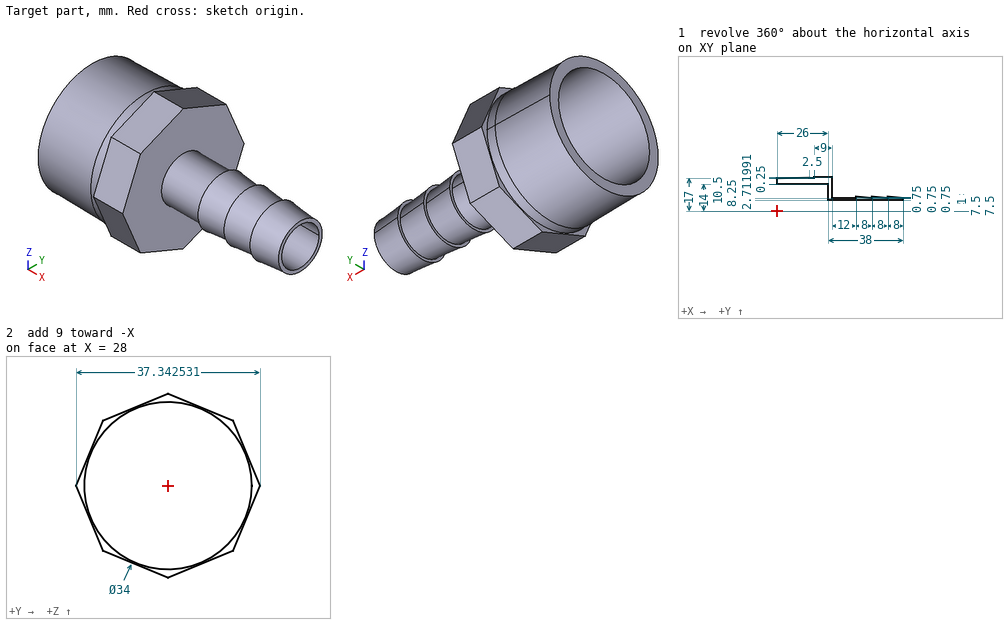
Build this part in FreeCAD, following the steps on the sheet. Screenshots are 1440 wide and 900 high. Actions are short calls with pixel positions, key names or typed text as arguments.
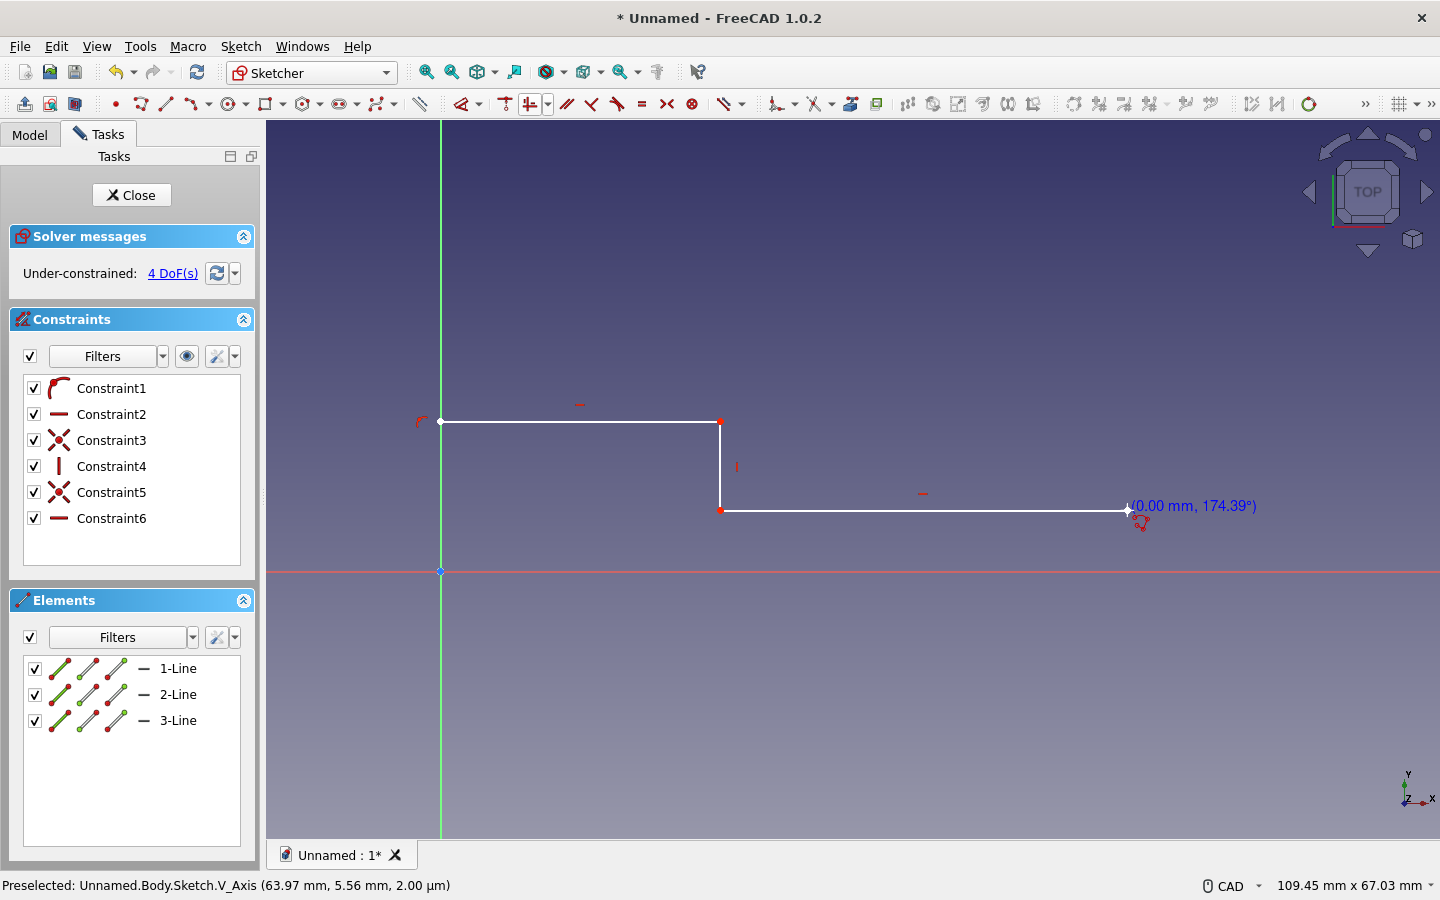
scroll(1127, 499, up, 2)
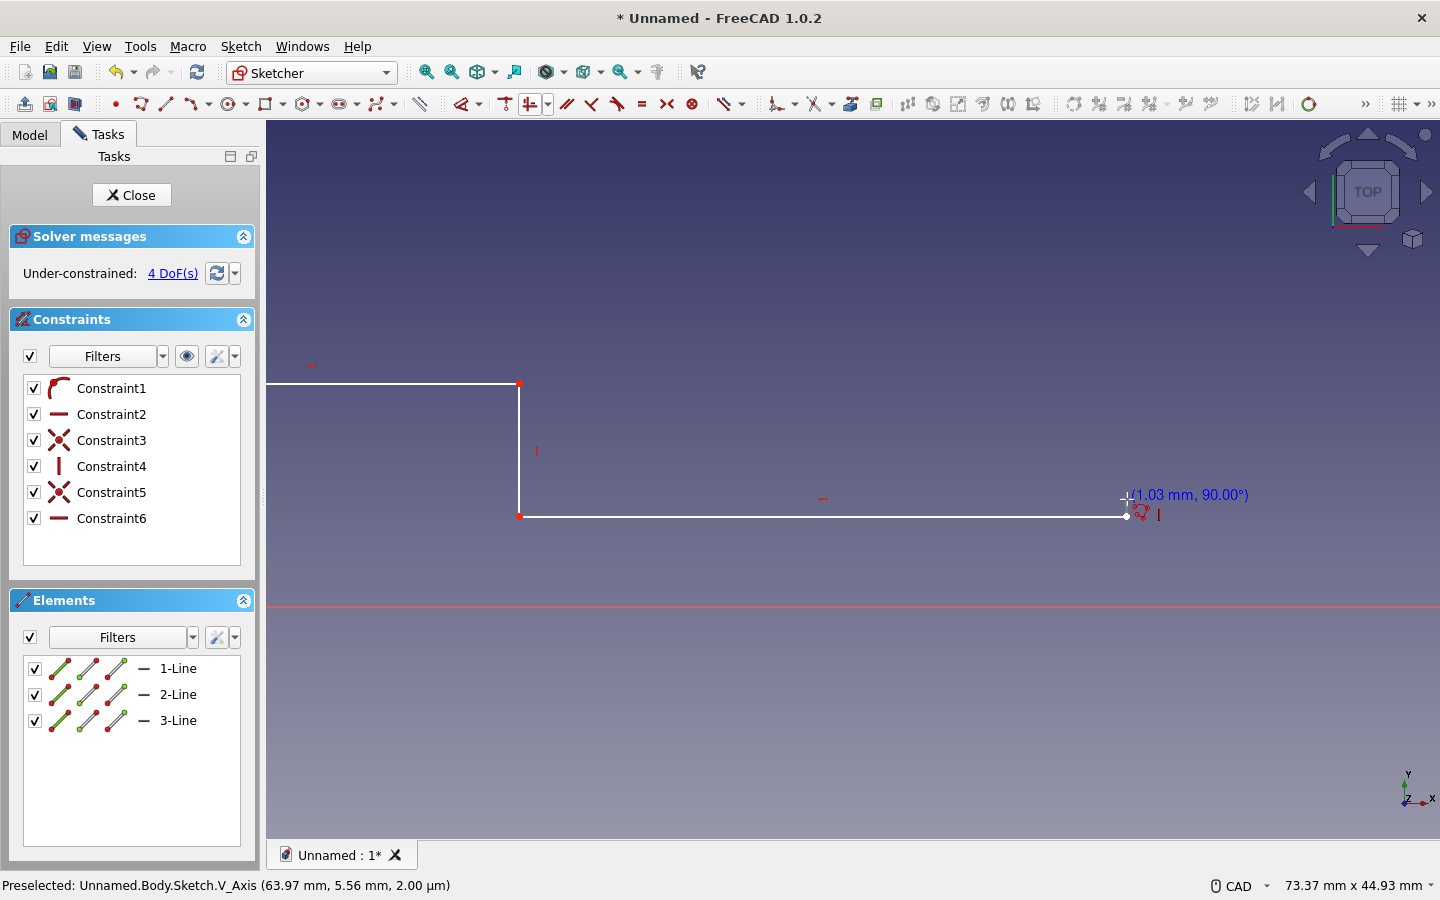
click(1127, 499)
click(999, 487)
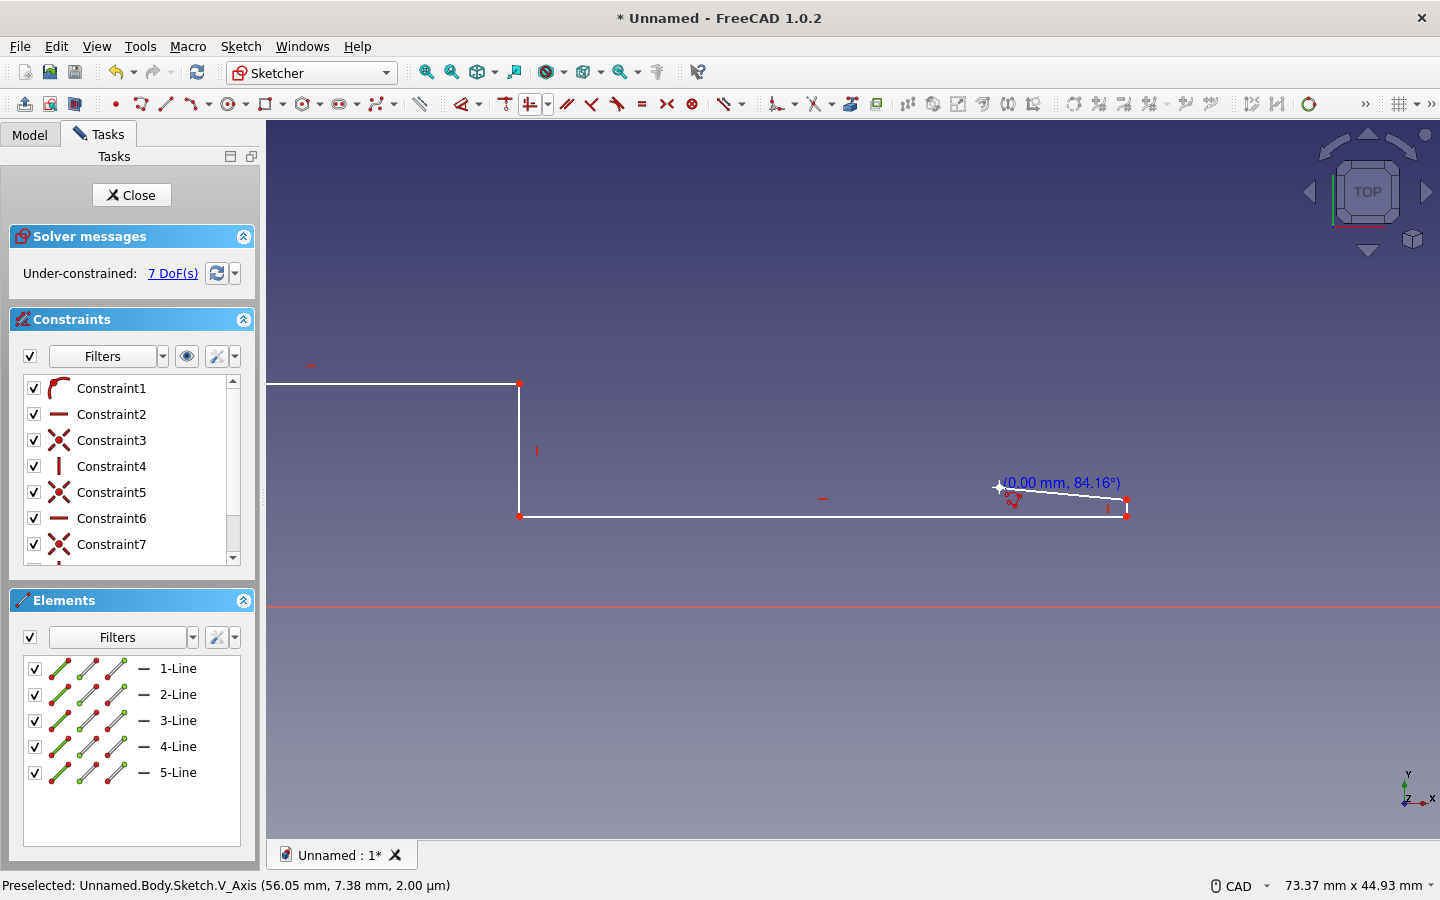
scroll(999, 499, up, 2)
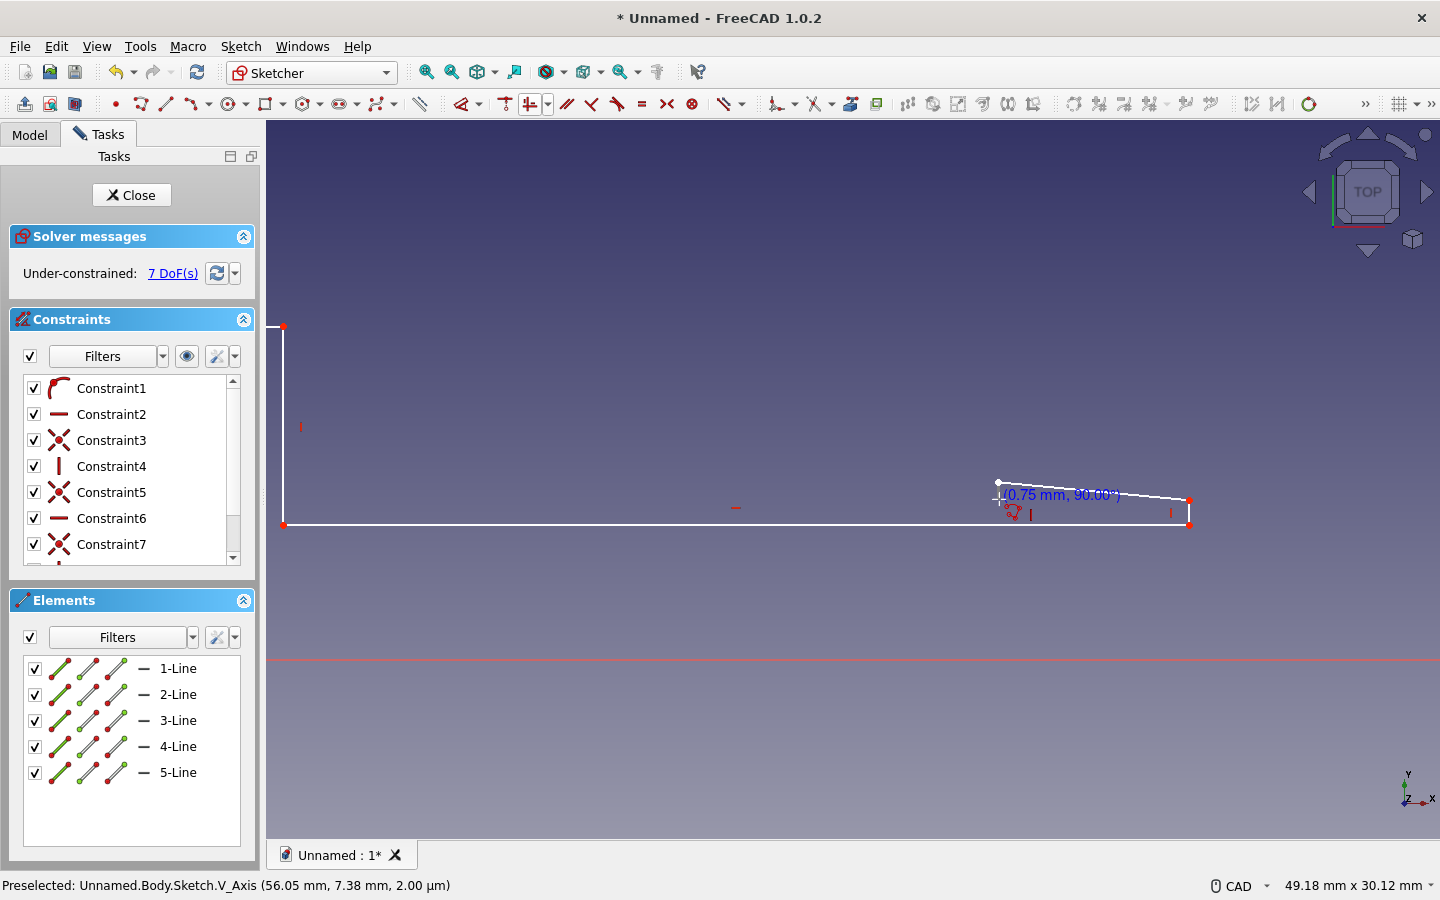
click(999, 499)
click(808, 481)
click(808, 499)
click(617, 481)
click(617, 499)
click(330, 499)
click(330, 248)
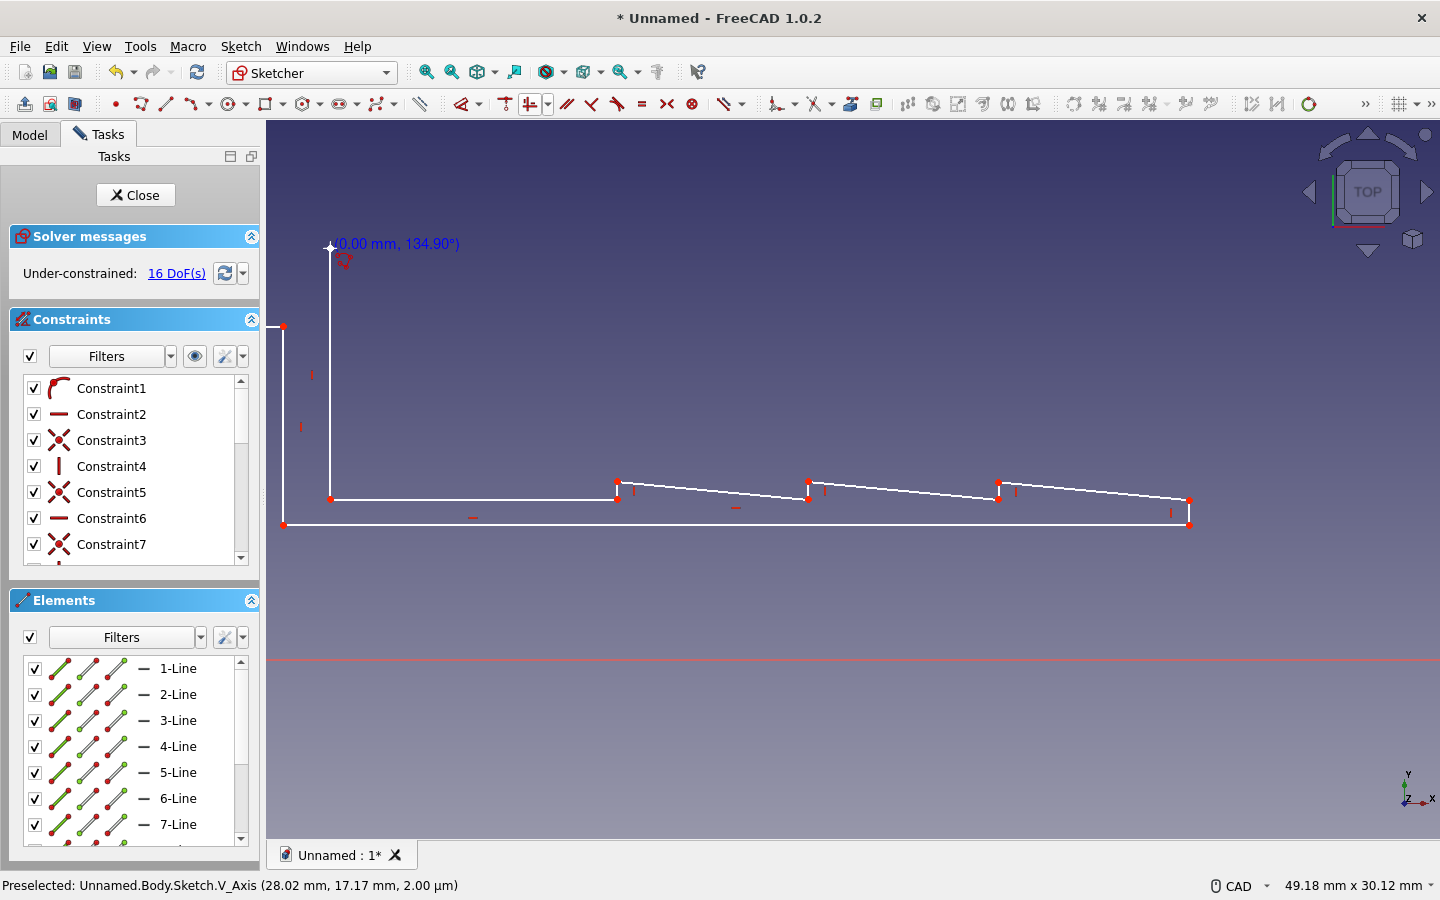
scroll(1077, 500, down, 4)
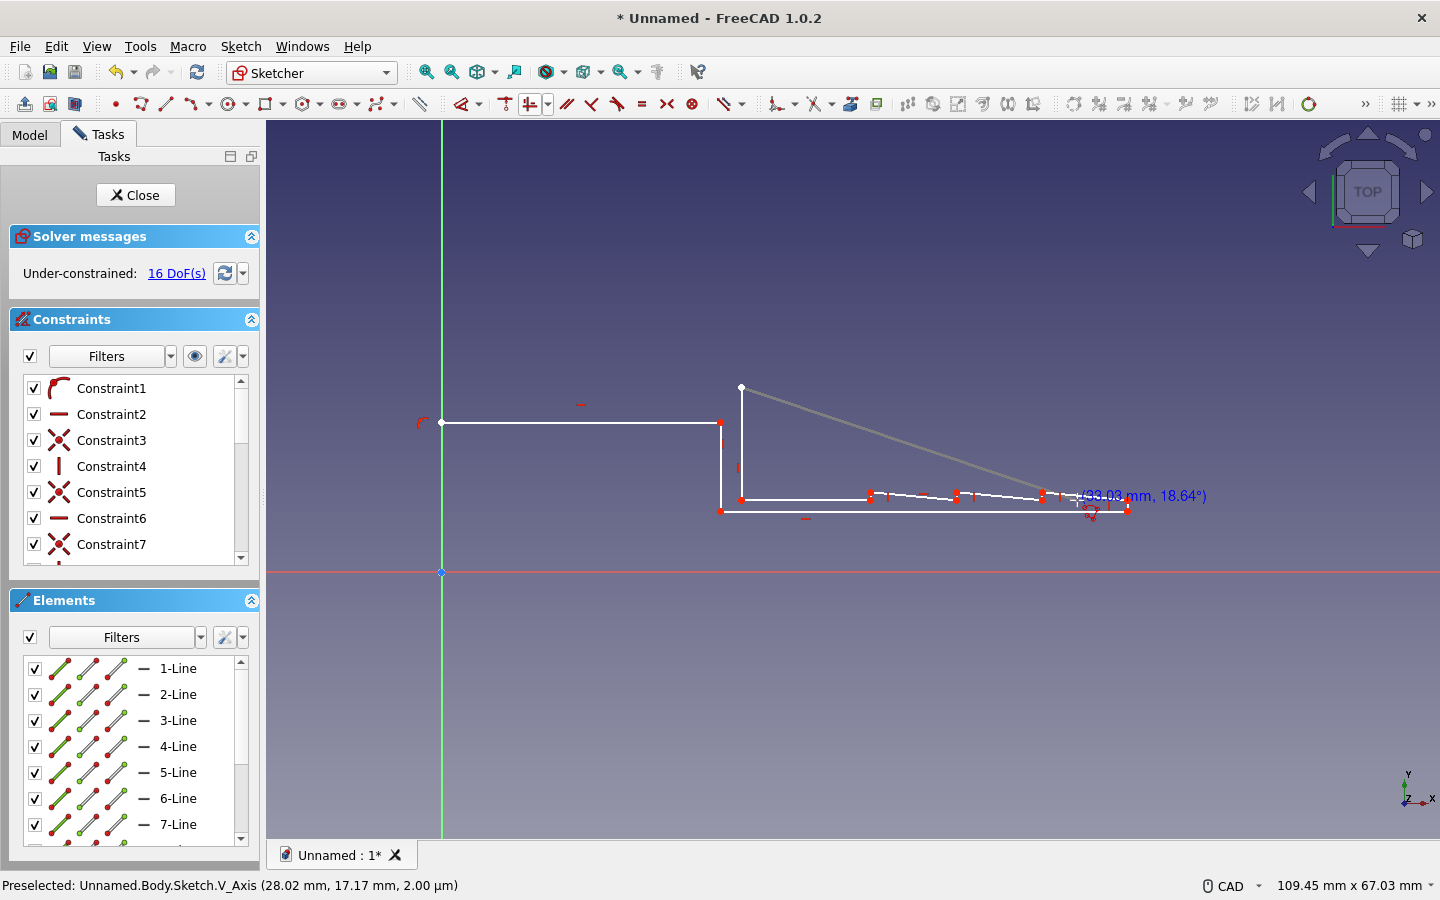
click(645, 387)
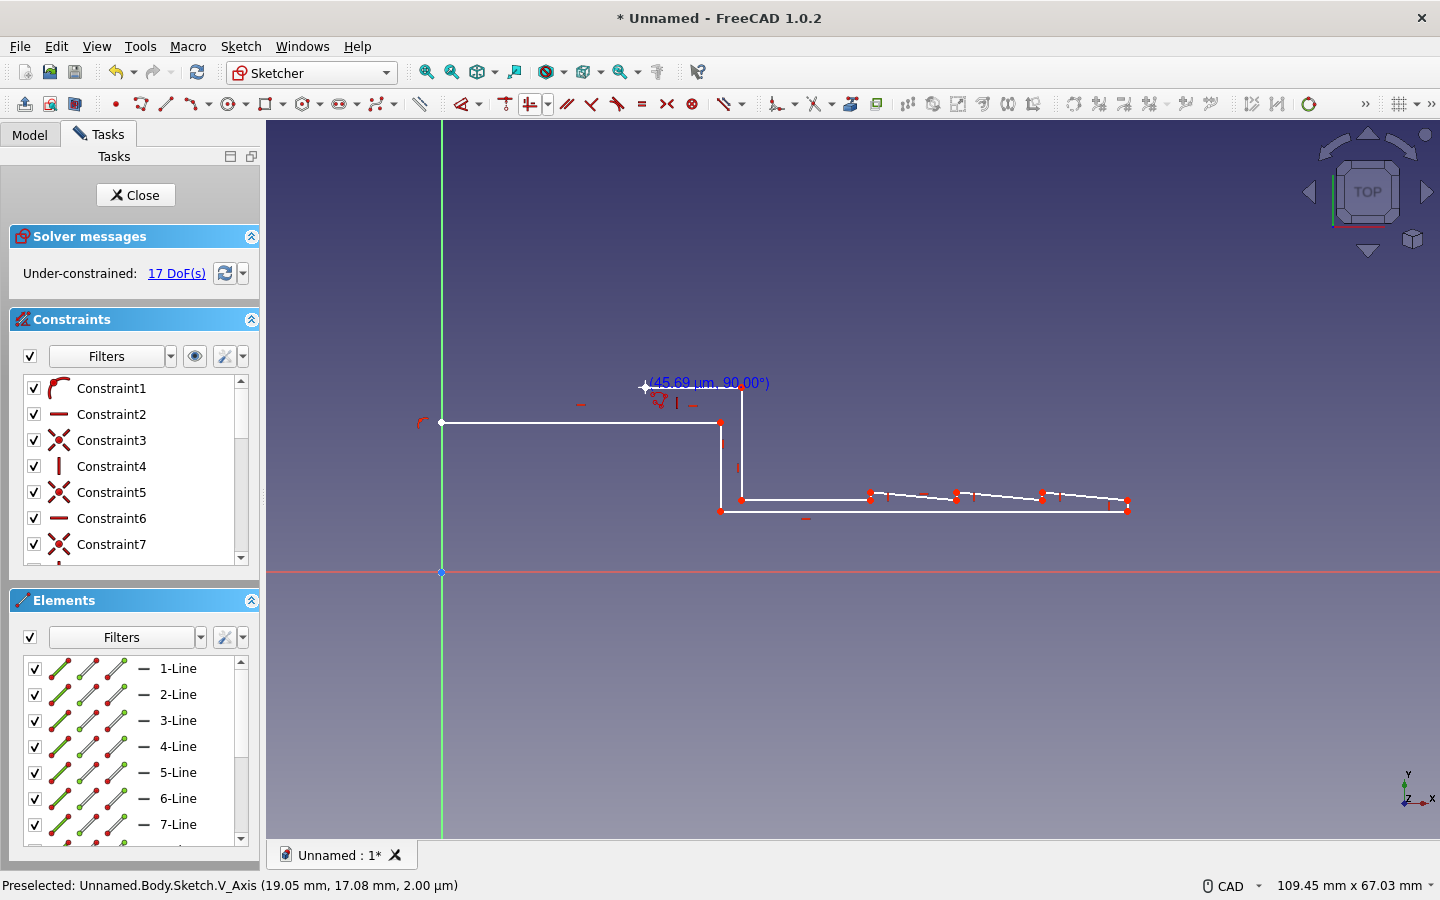
scroll(645, 390, up, 9)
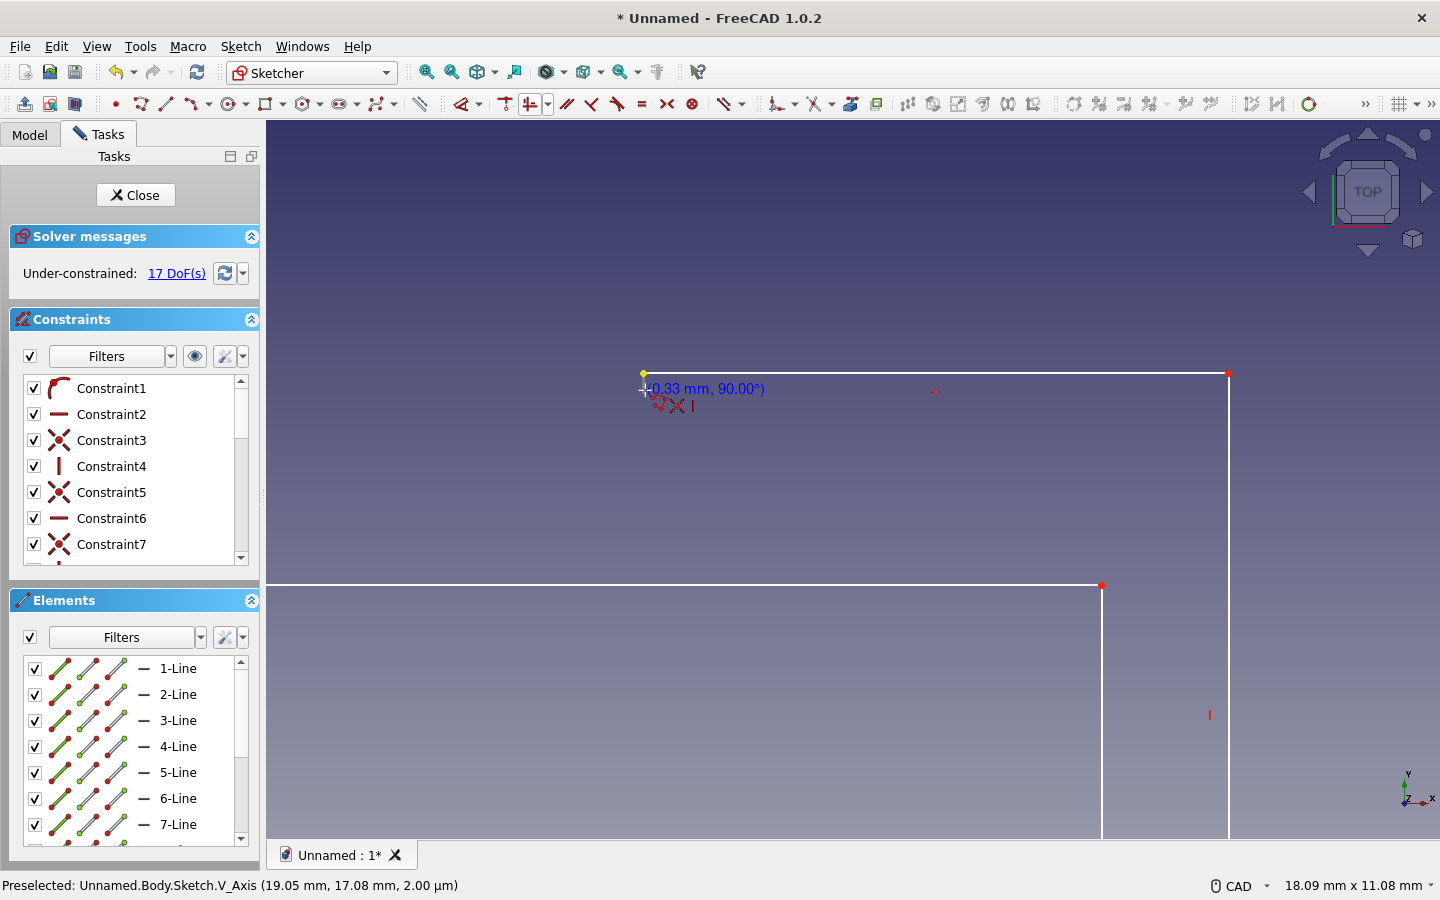
click(643, 387)